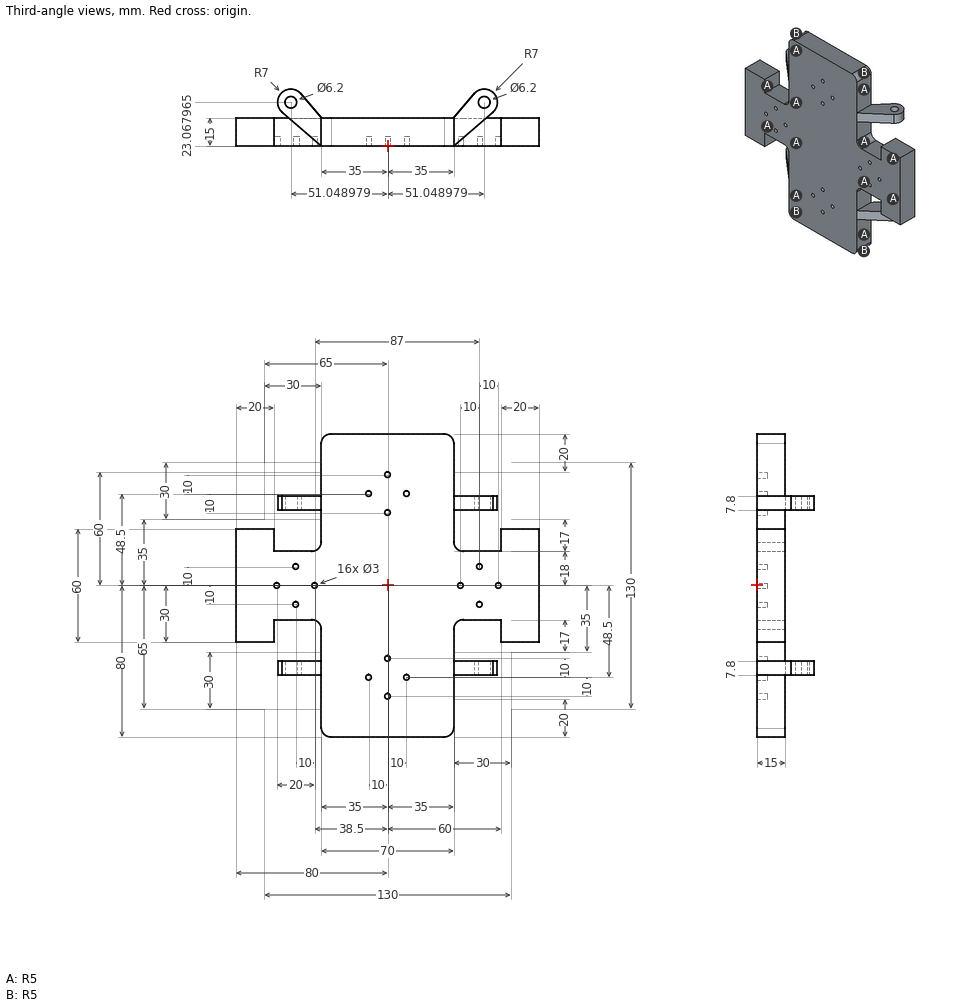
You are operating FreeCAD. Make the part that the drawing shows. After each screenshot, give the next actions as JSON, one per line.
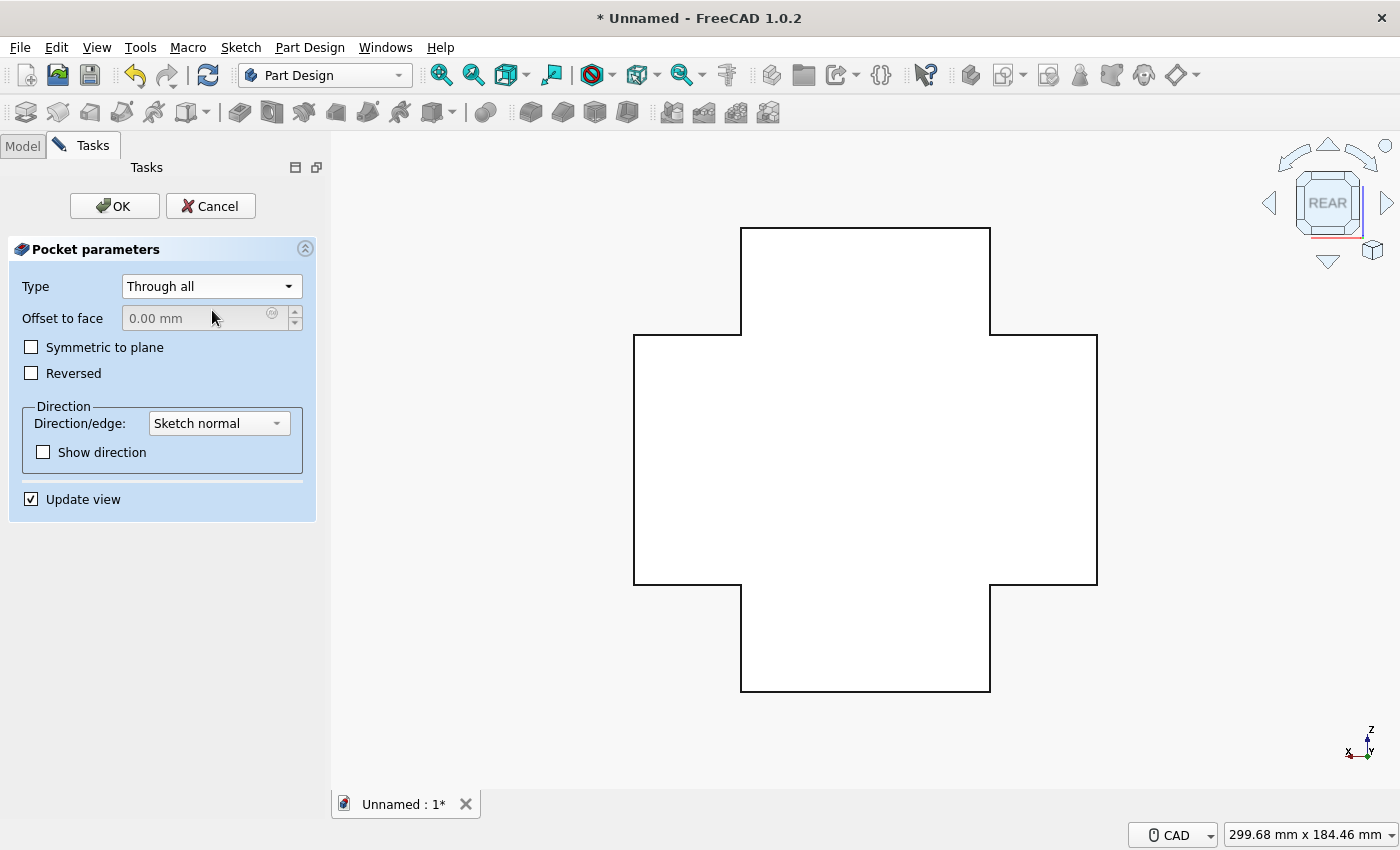
{"action": "left_click", "coordinate": [115, 206]}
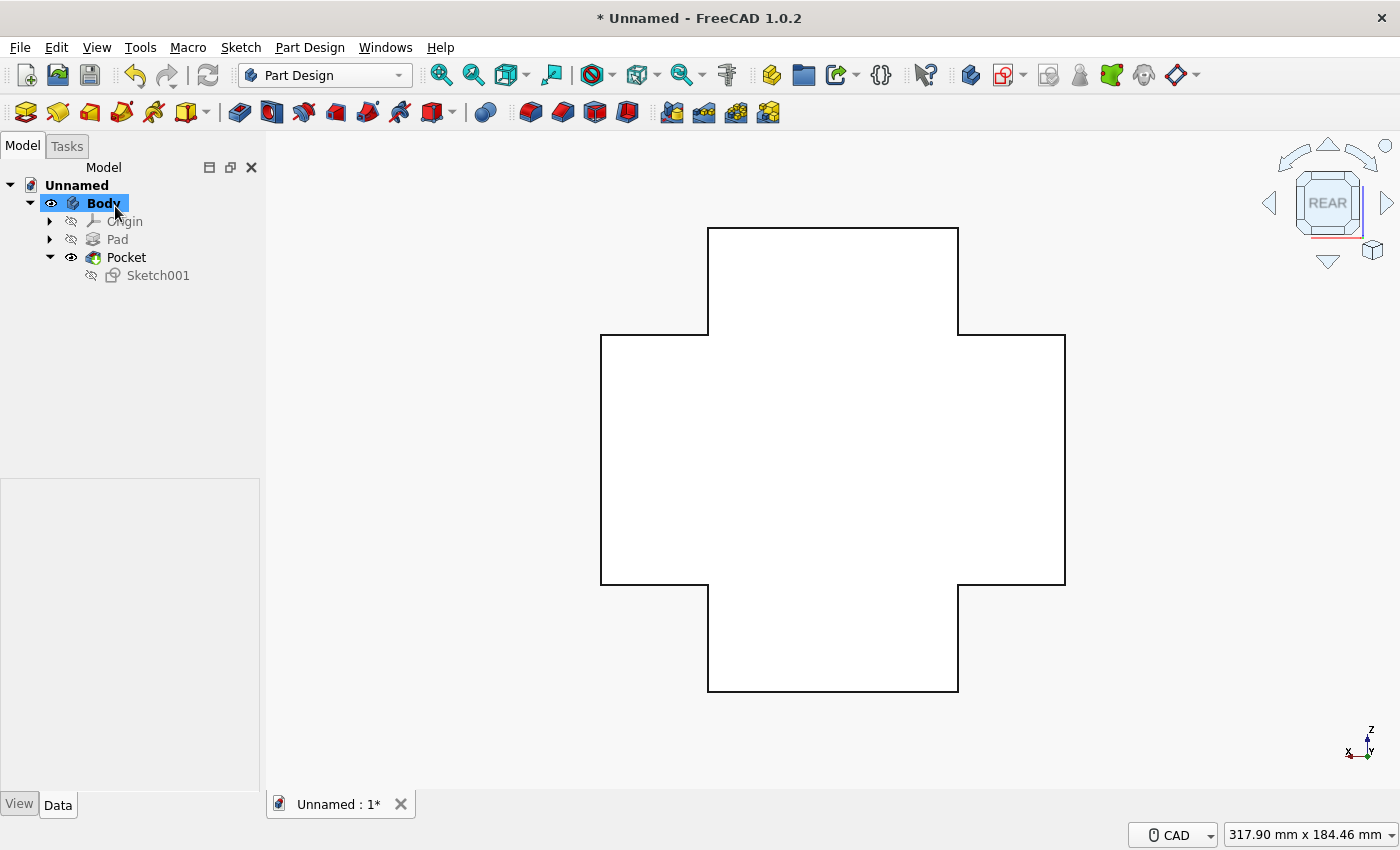
{"action": "left_click", "coordinate": [50, 221]}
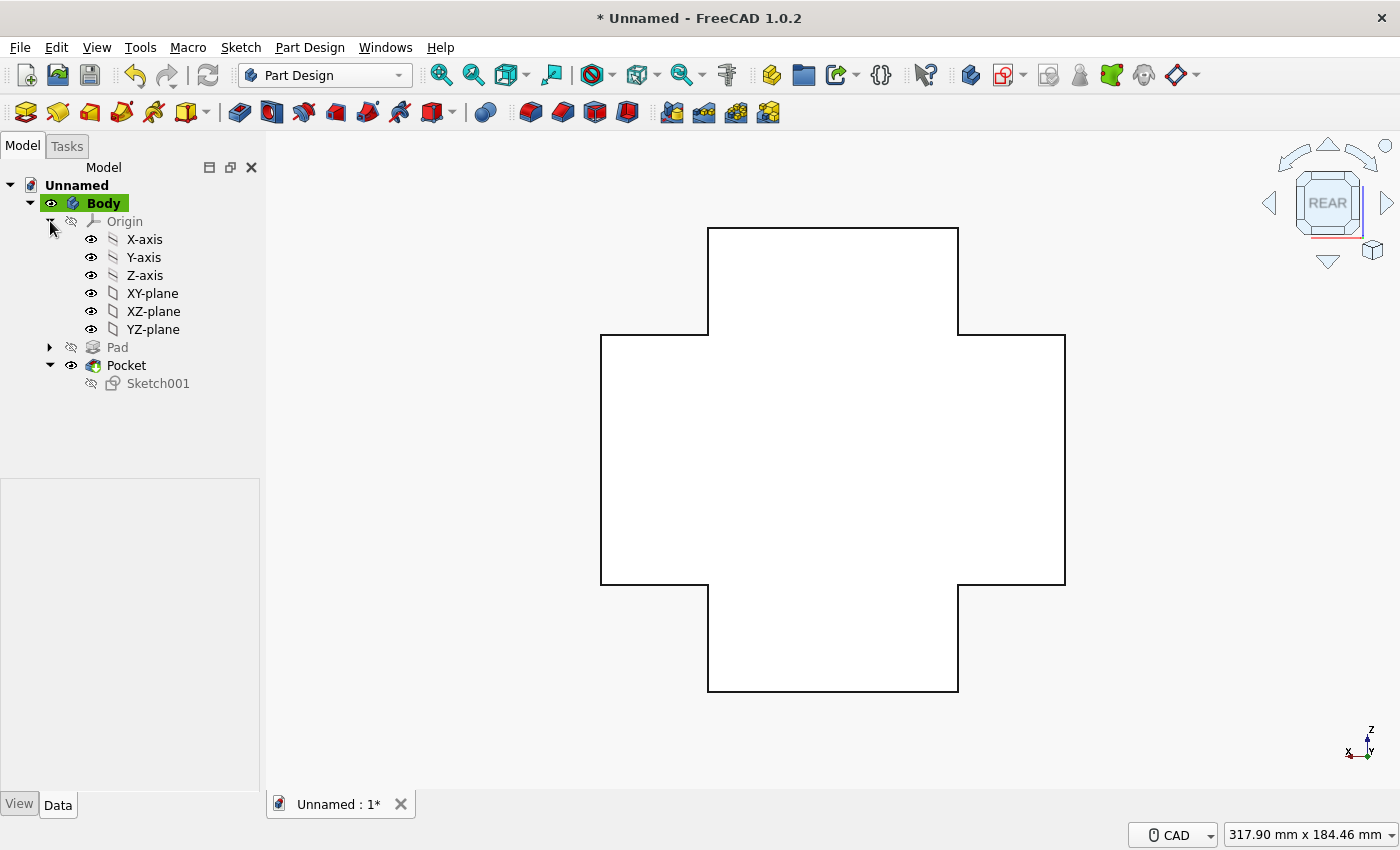
{"action": "left_click", "coordinate": [136, 311]}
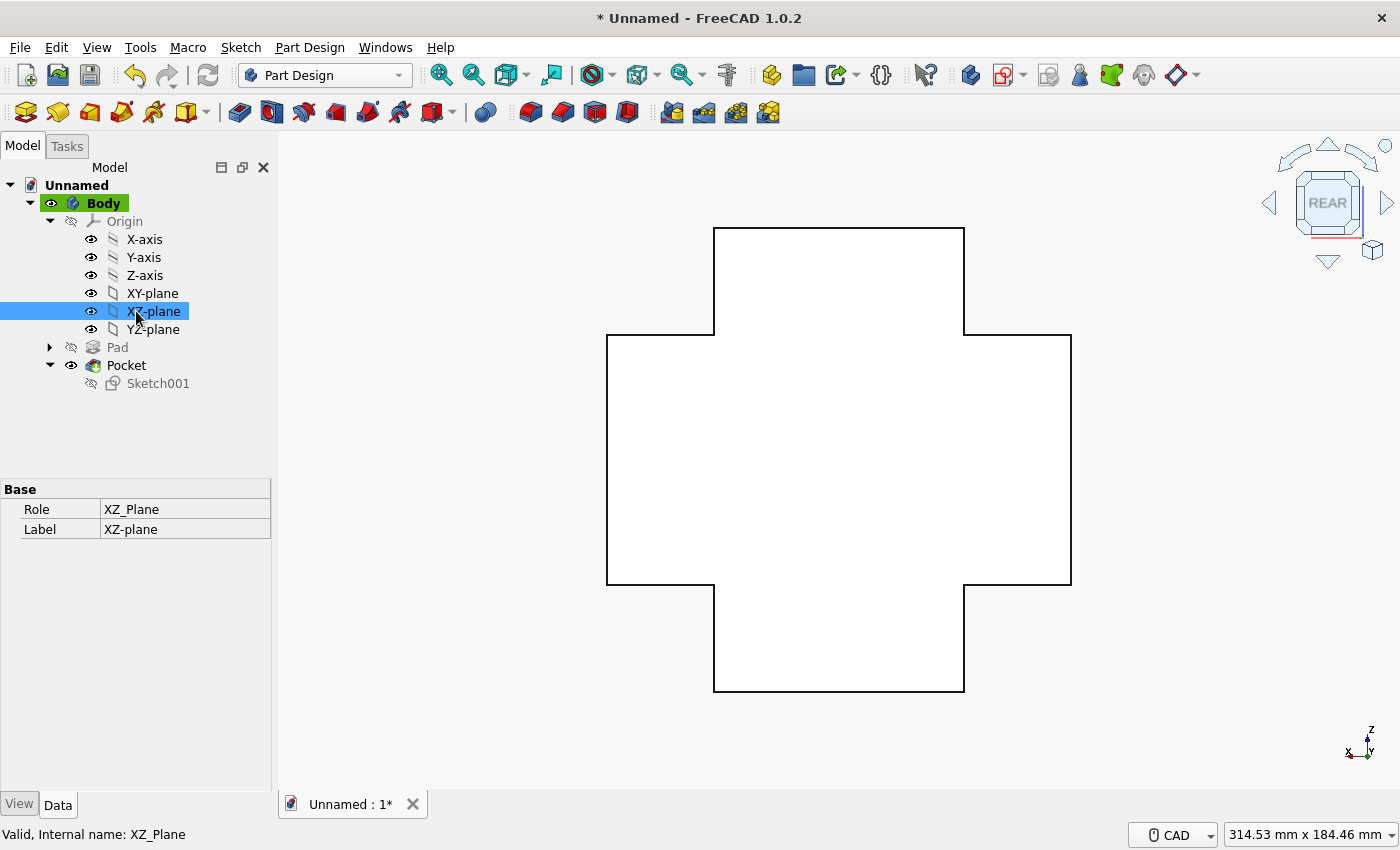
{"action": "left_click", "coordinate": [1176, 76]}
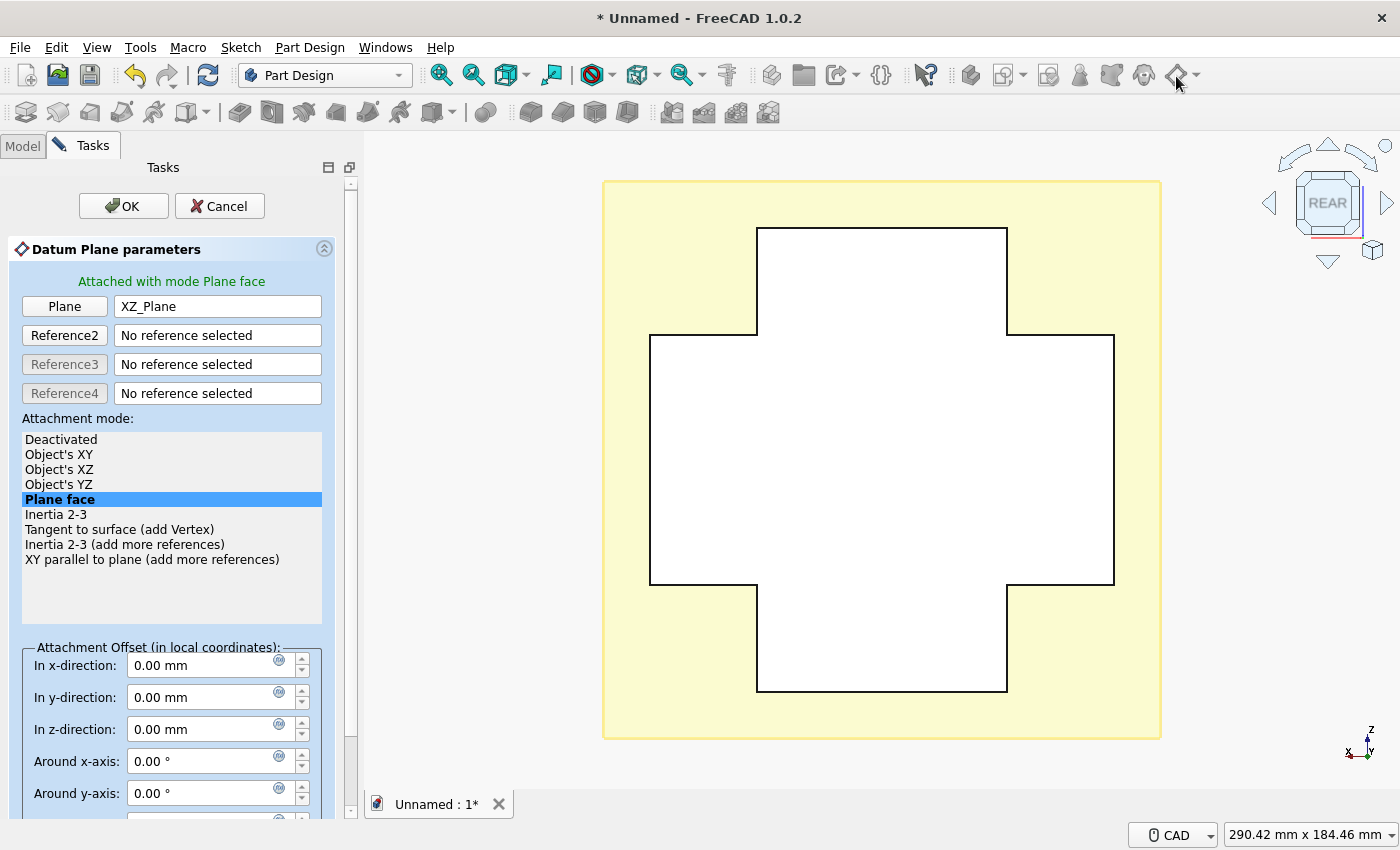
{"action": "triple_click", "coordinate": [210, 729]}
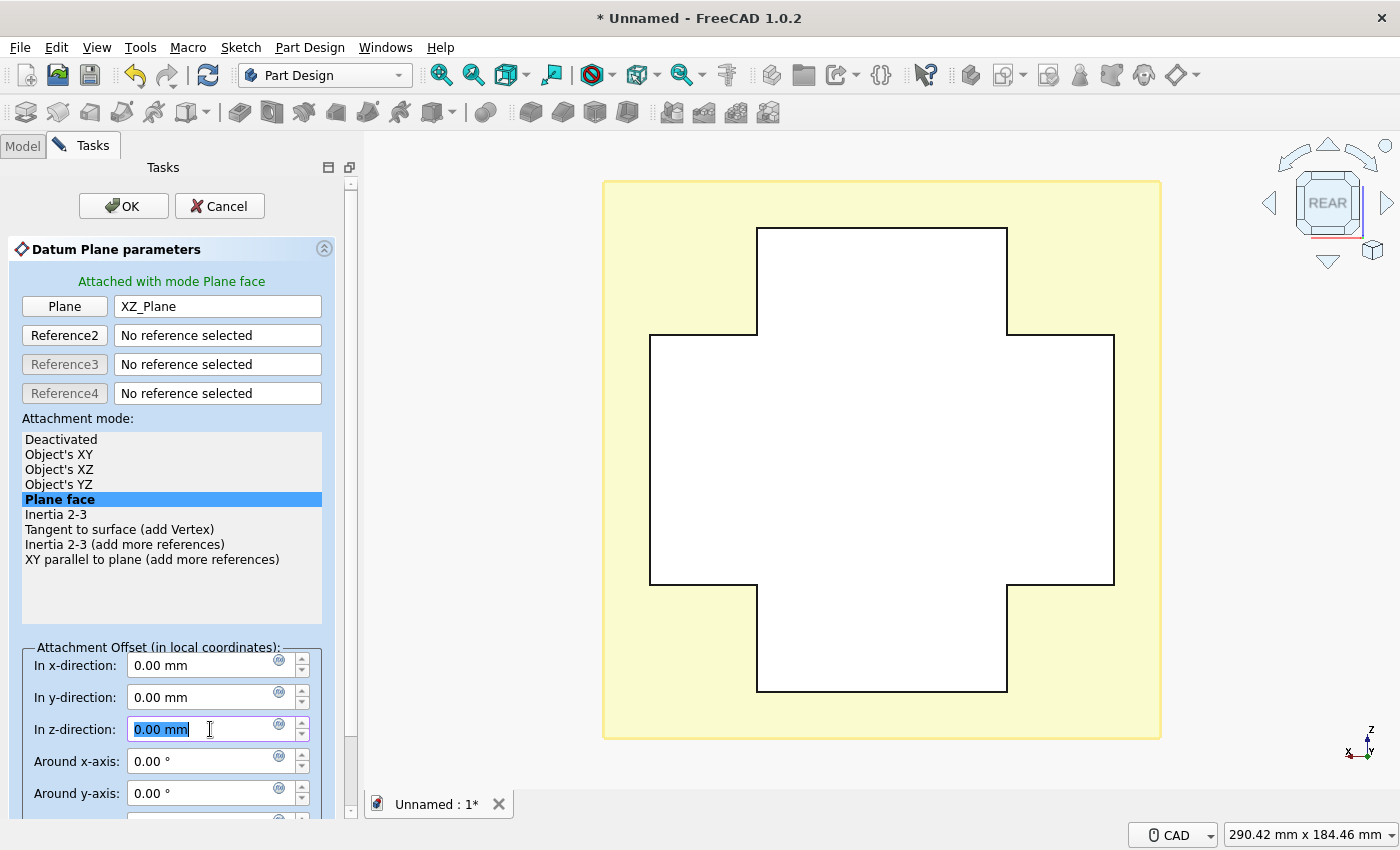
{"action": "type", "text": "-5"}
{"action": "key", "text": "Tab"}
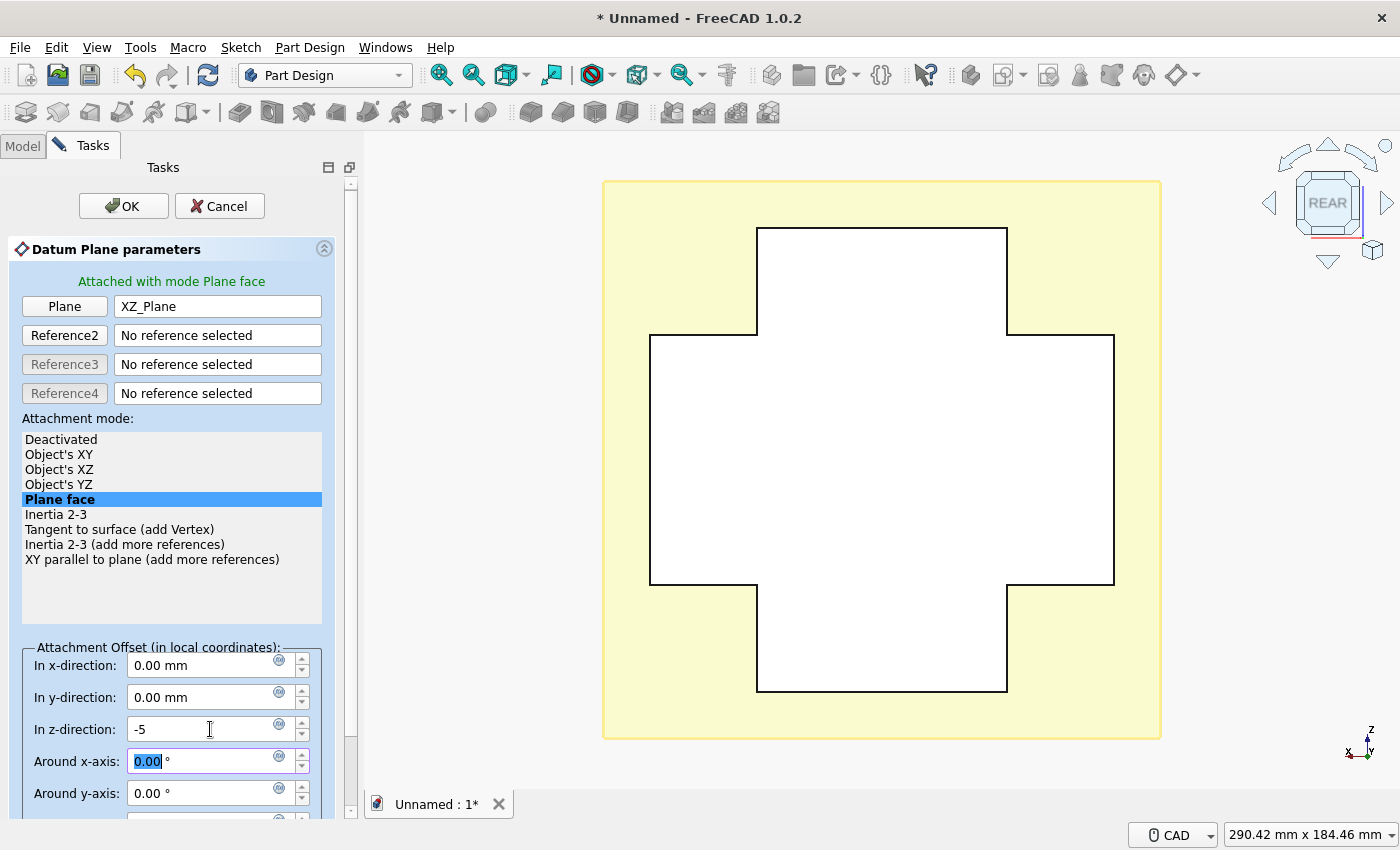
{"action": "left_click", "coordinate": [124, 206]}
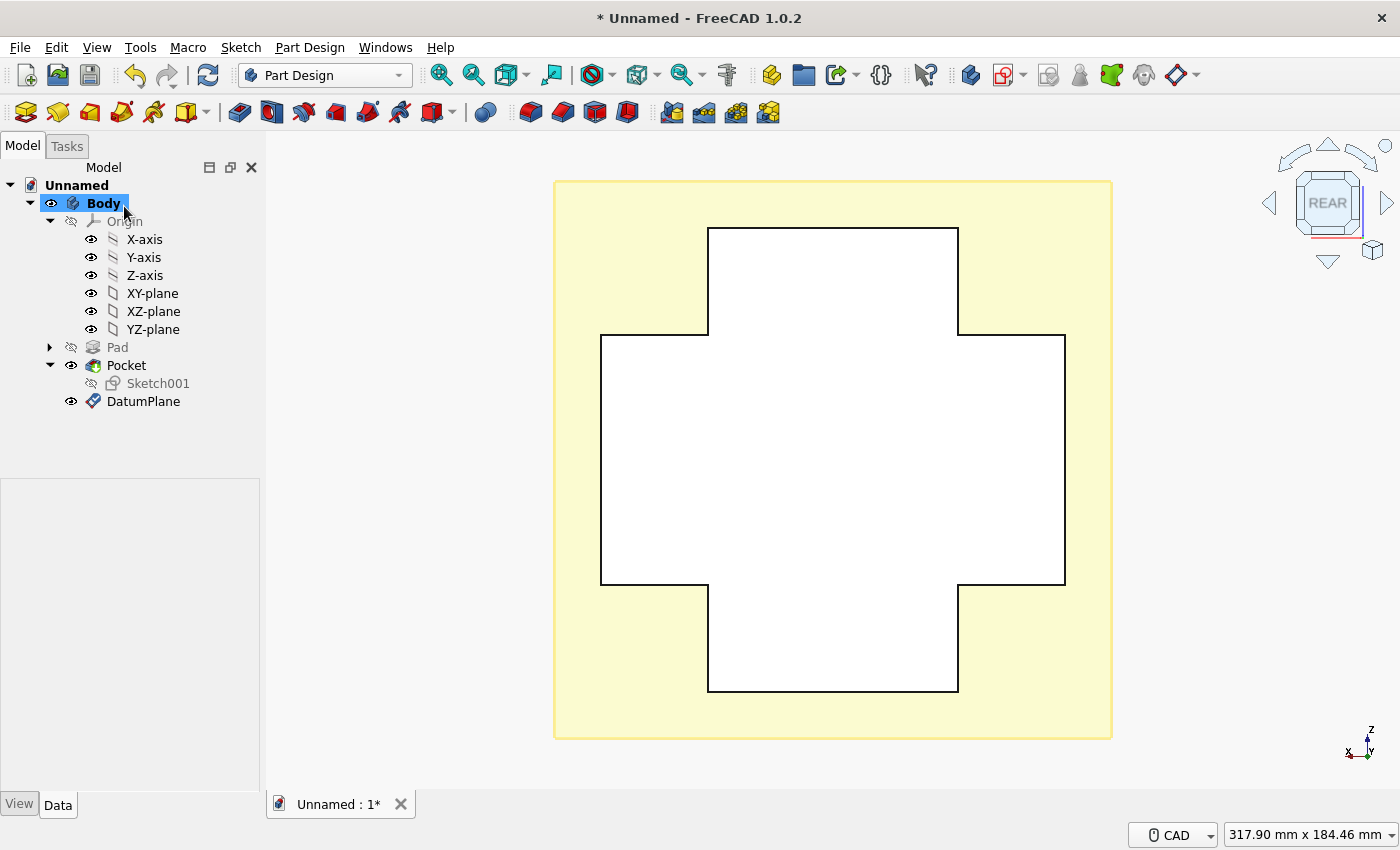
{"action": "left_click", "coordinate": [116, 401]}